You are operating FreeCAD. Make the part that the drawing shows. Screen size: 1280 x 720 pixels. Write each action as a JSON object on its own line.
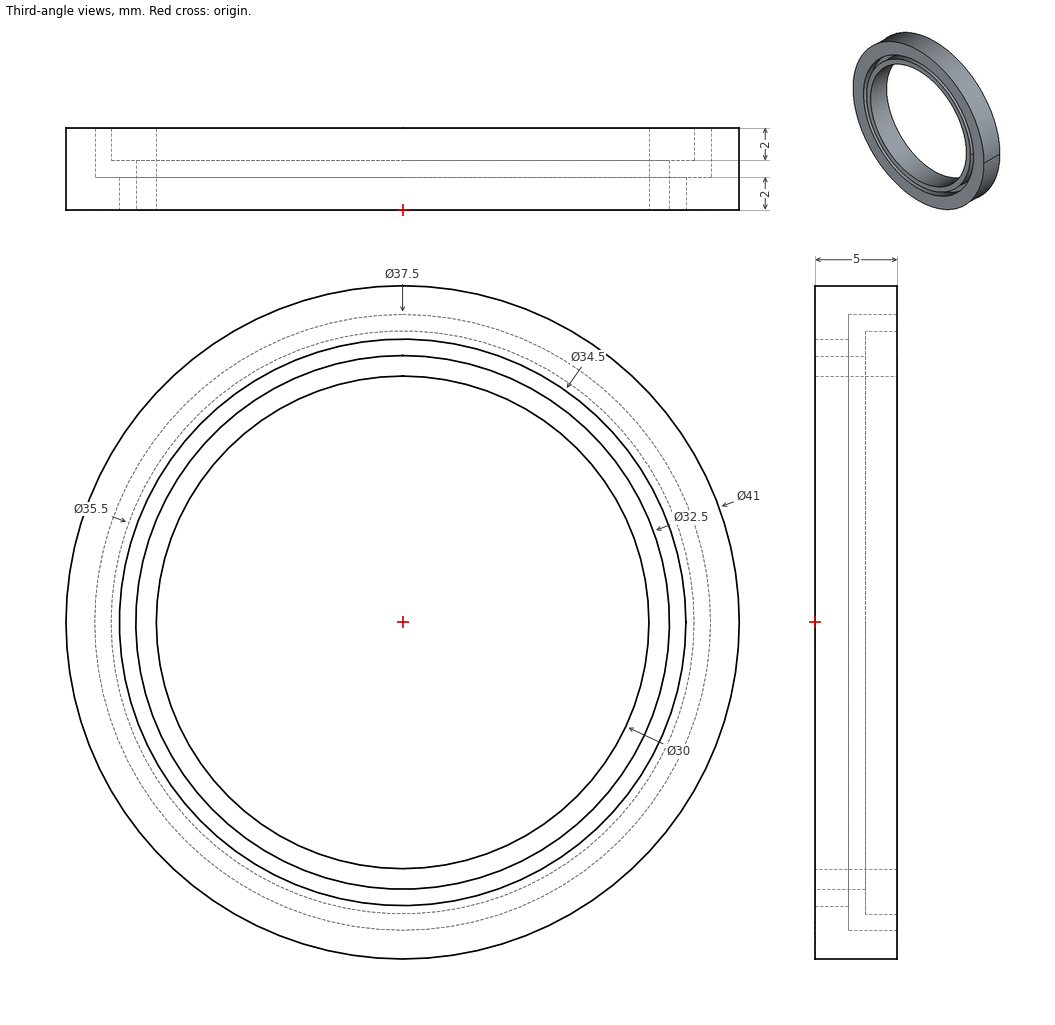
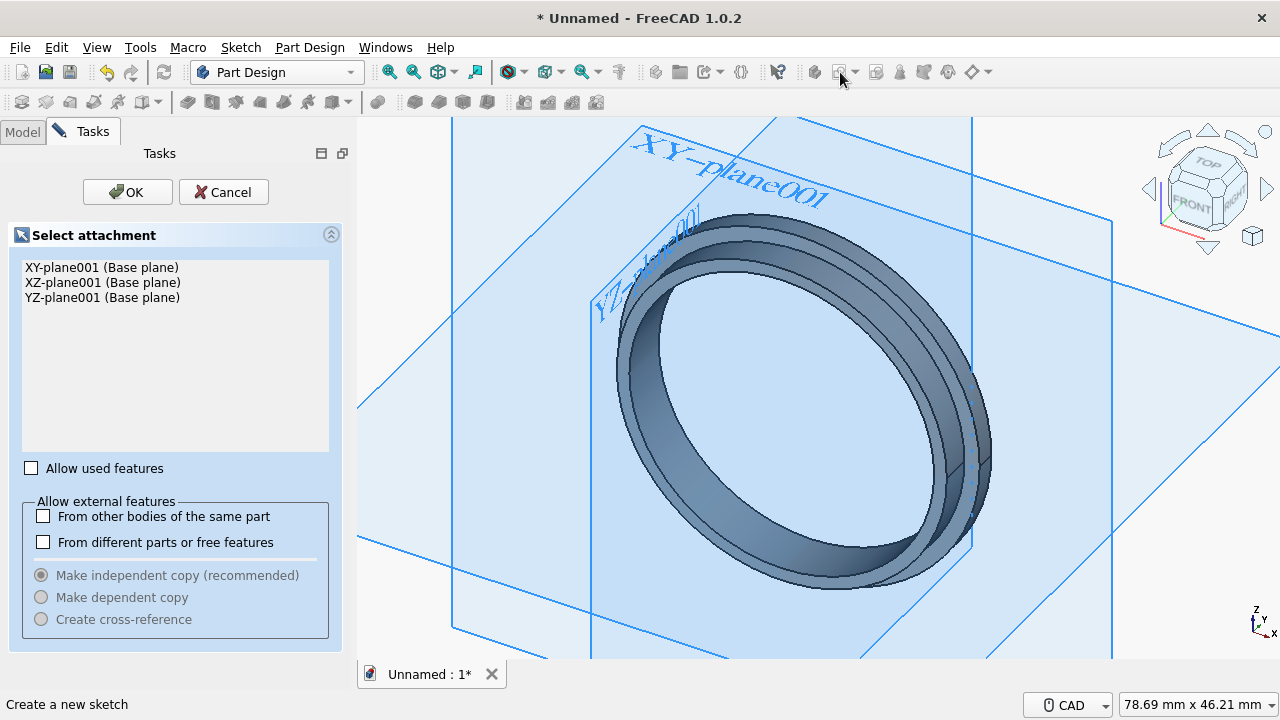
{"action": "left_click", "coordinate": [82, 282]}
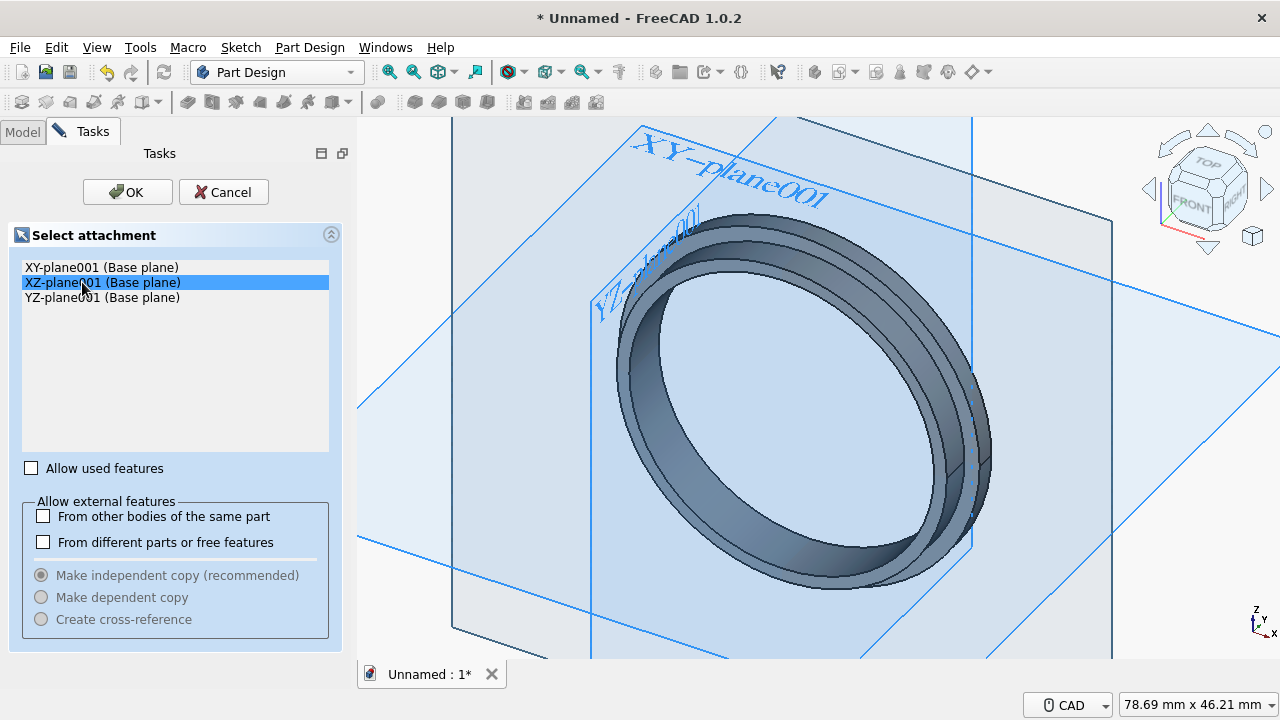
{"action": "left_click", "coordinate": [128, 192]}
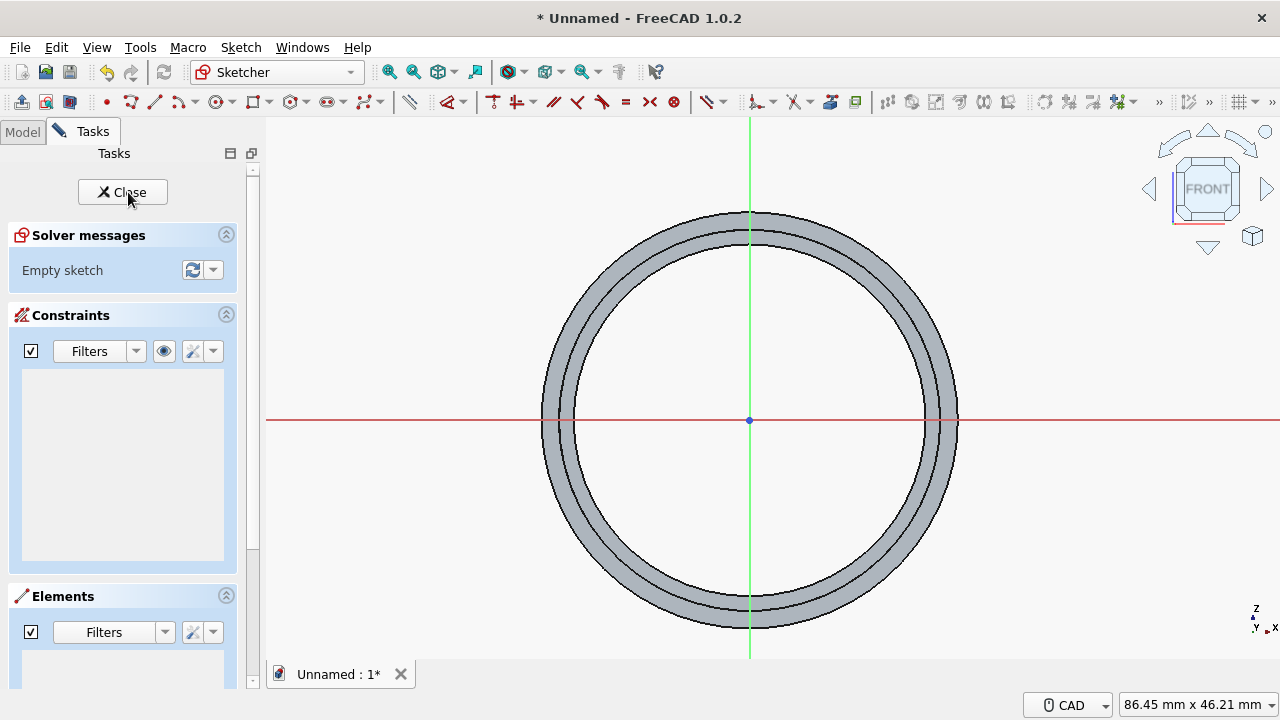
{"action": "scroll", "coordinate": [613, 322], "scroll_direction": "down", "scroll_amount": 2}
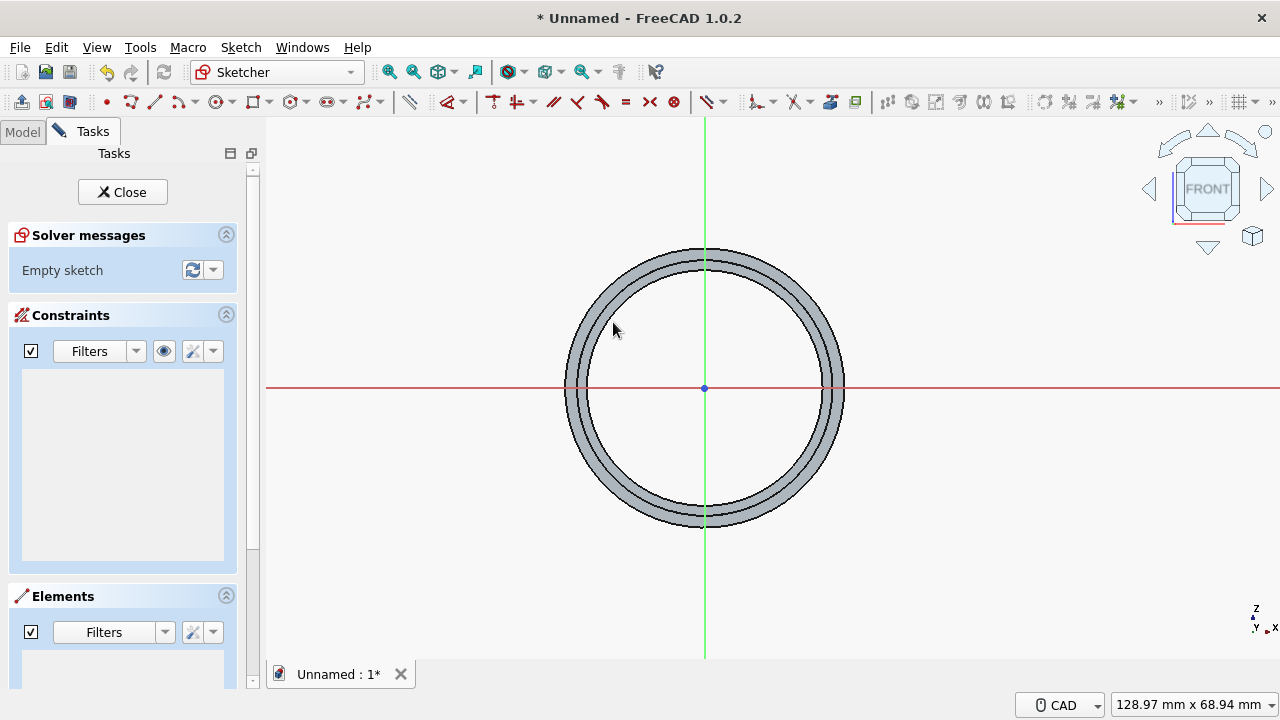
{"action": "key", "text": "g c"}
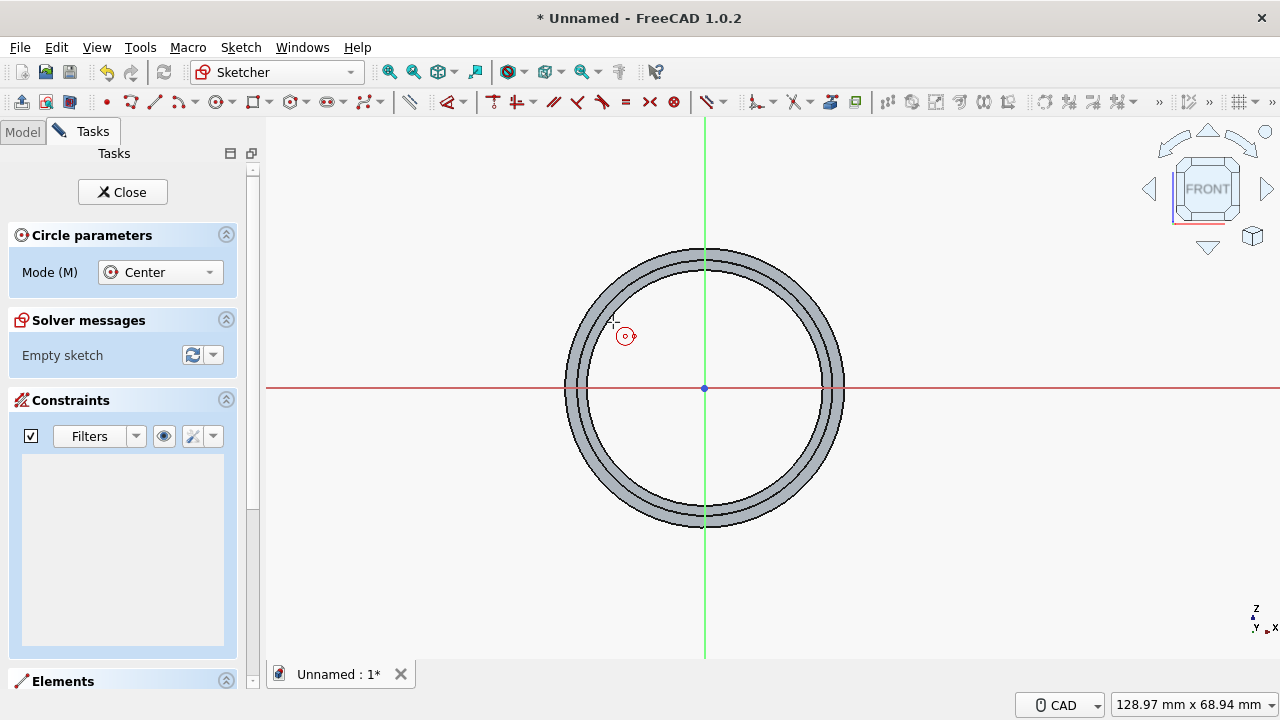
{"action": "left_click", "coordinate": [705, 388]}
{"action": "mouse_move", "coordinate": [819, 274]}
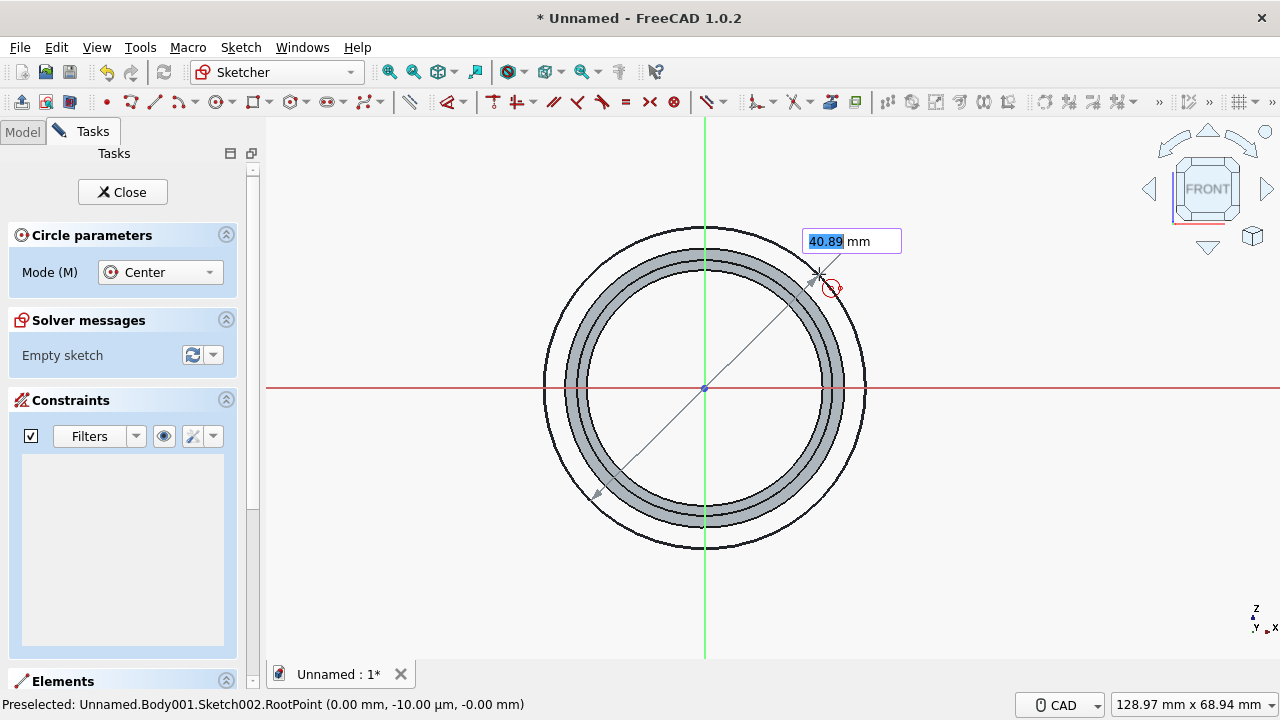
{"action": "type", "text": "41"}
{"action": "key", "text": "Return"}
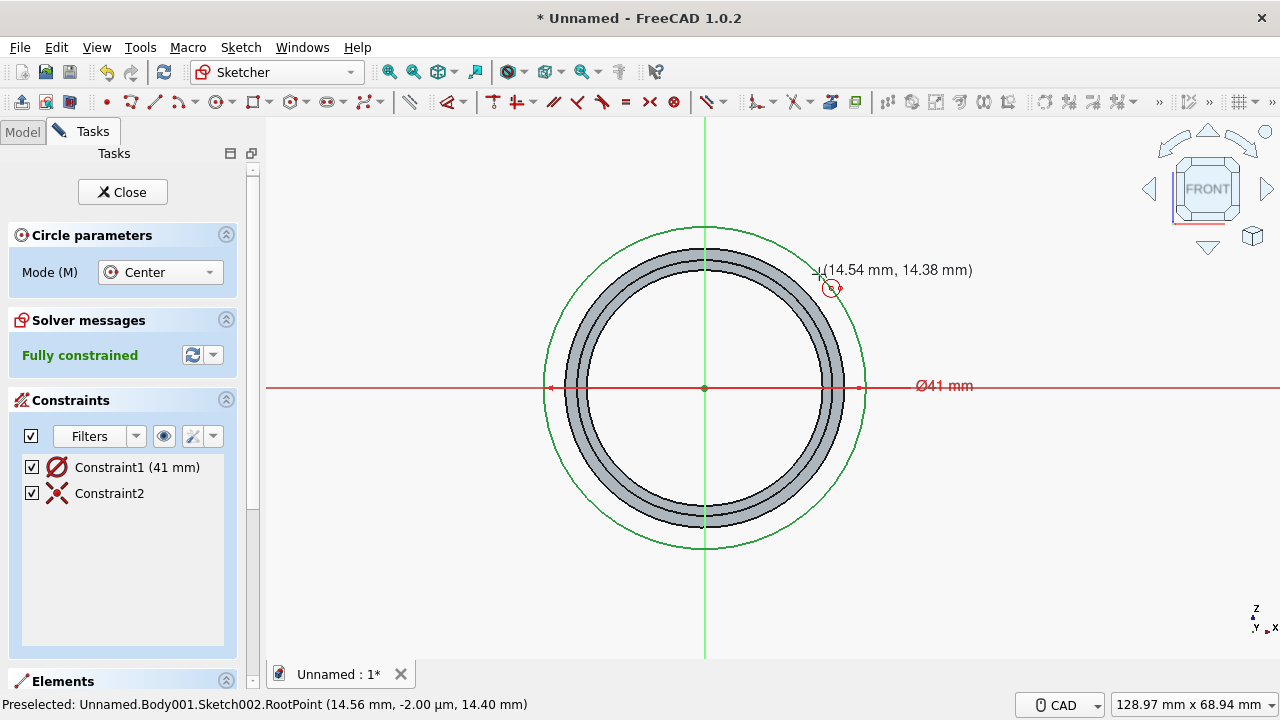
{"action": "left_click", "coordinate": [705, 388]}
{"action": "mouse_move", "coordinate": [809, 284]}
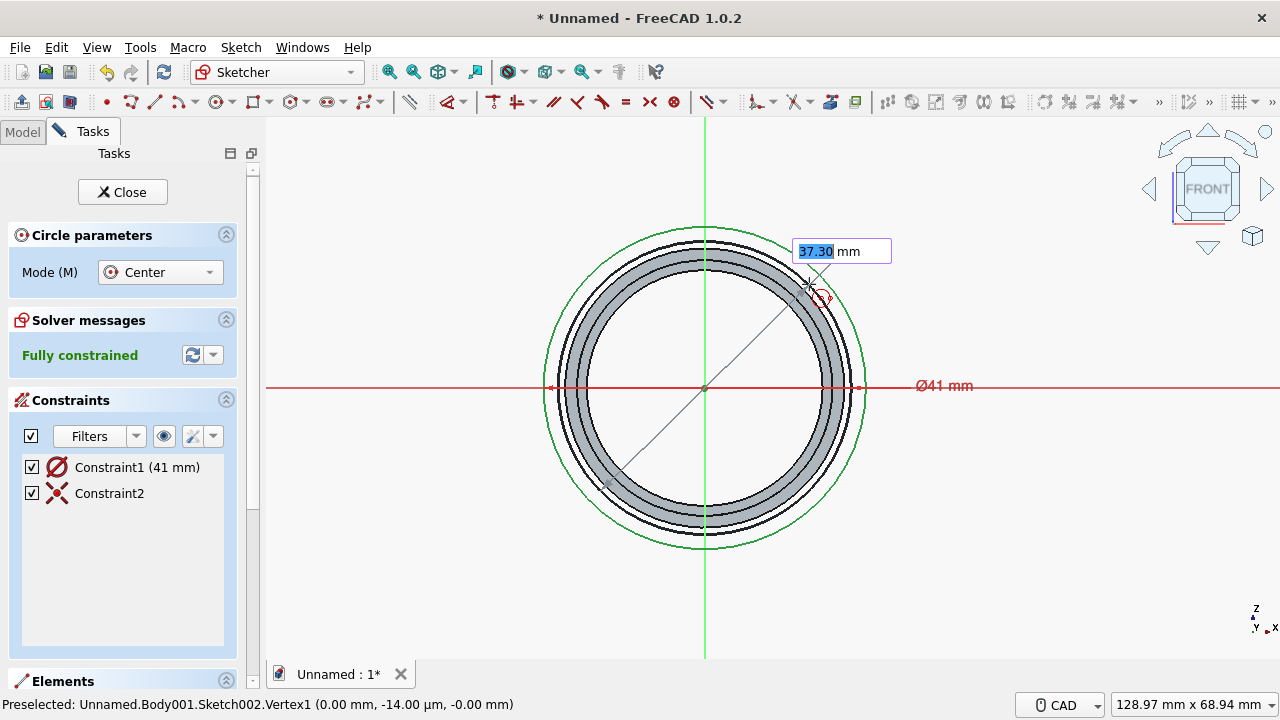
{"action": "type", "text": "37.5"}
{"action": "key", "text": "Return"}
{"action": "key", "text": "Escape"}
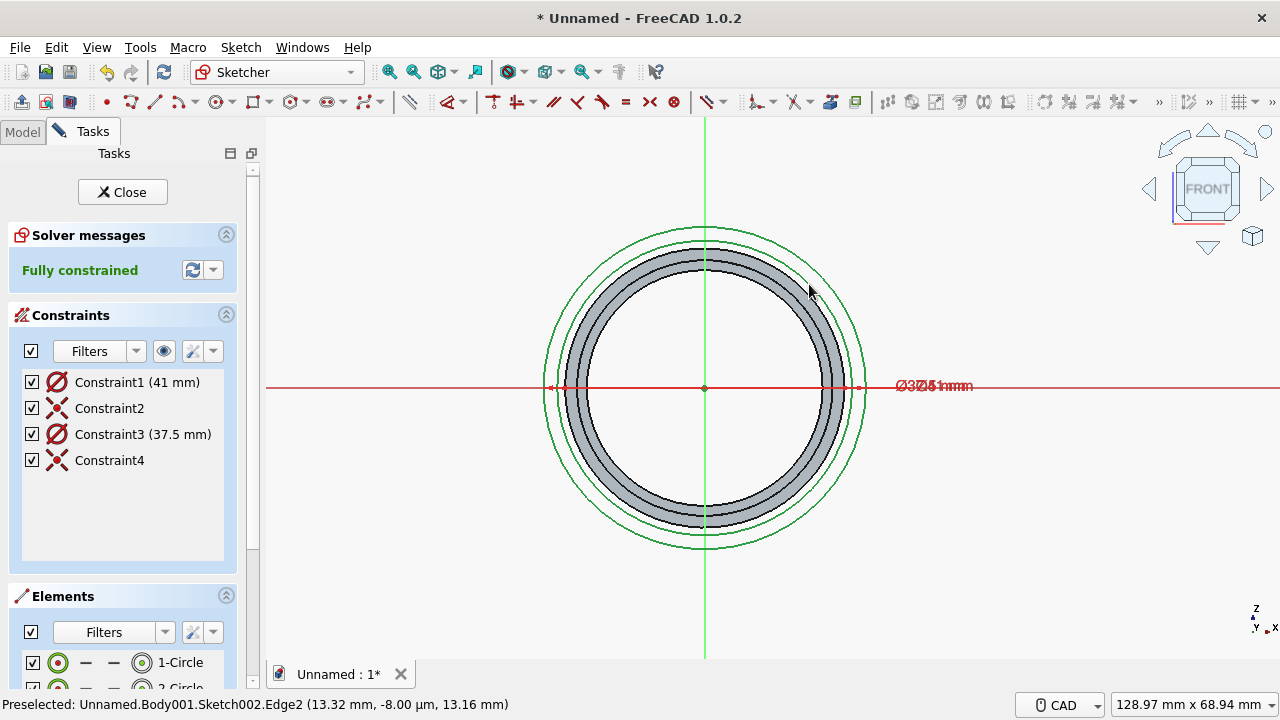
{"action": "left_click", "coordinate": [123, 192]}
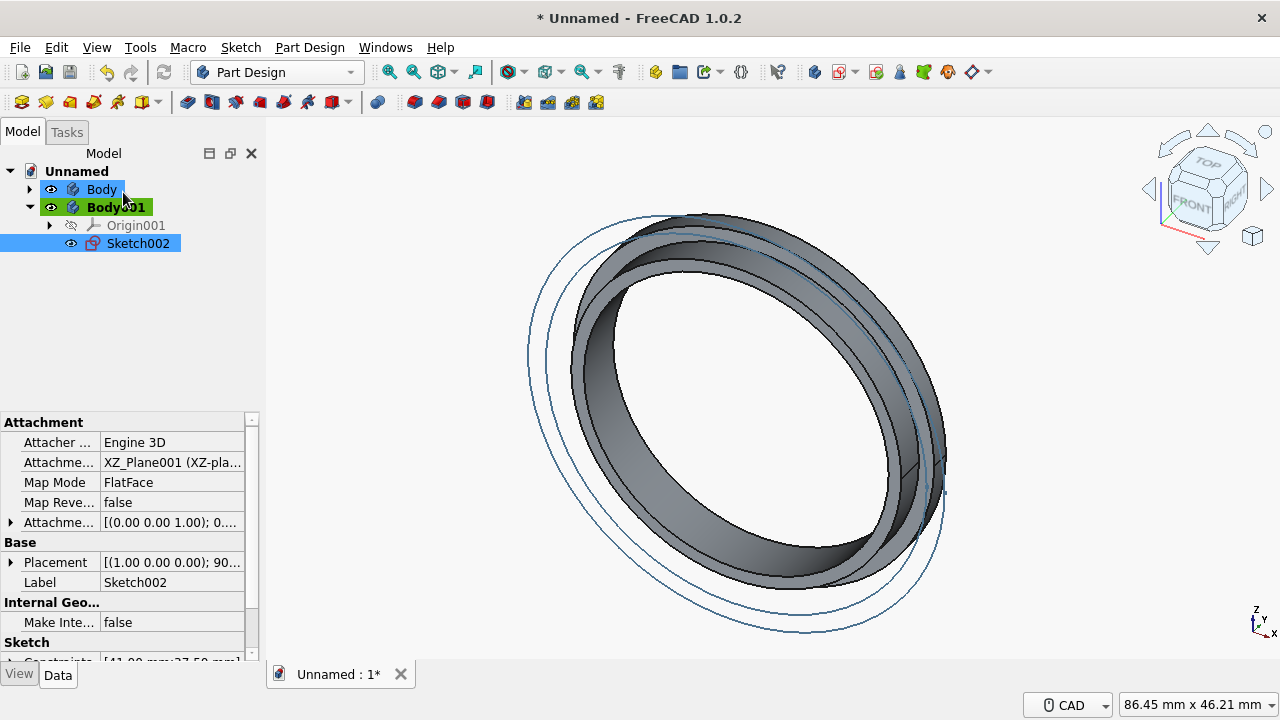
{"action": "left_click", "coordinate": [22, 102]}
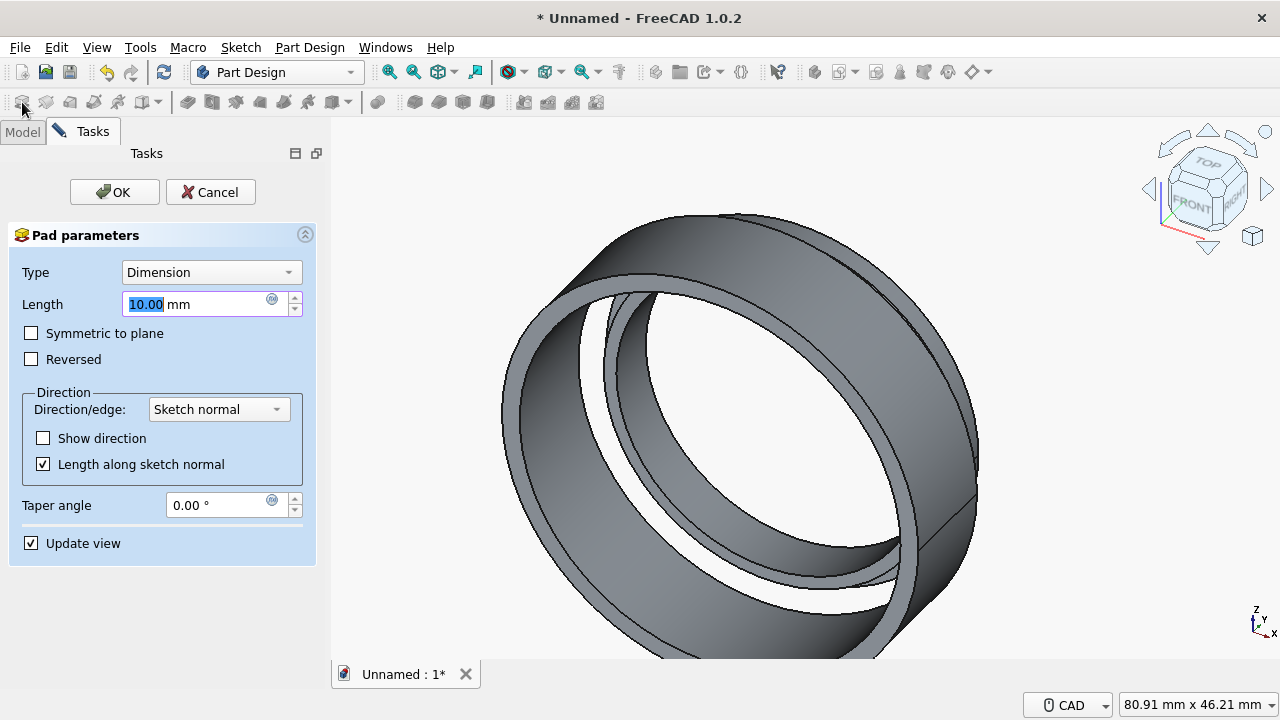
{"action": "type", "text": "5"}
{"action": "key", "text": "Tab"}